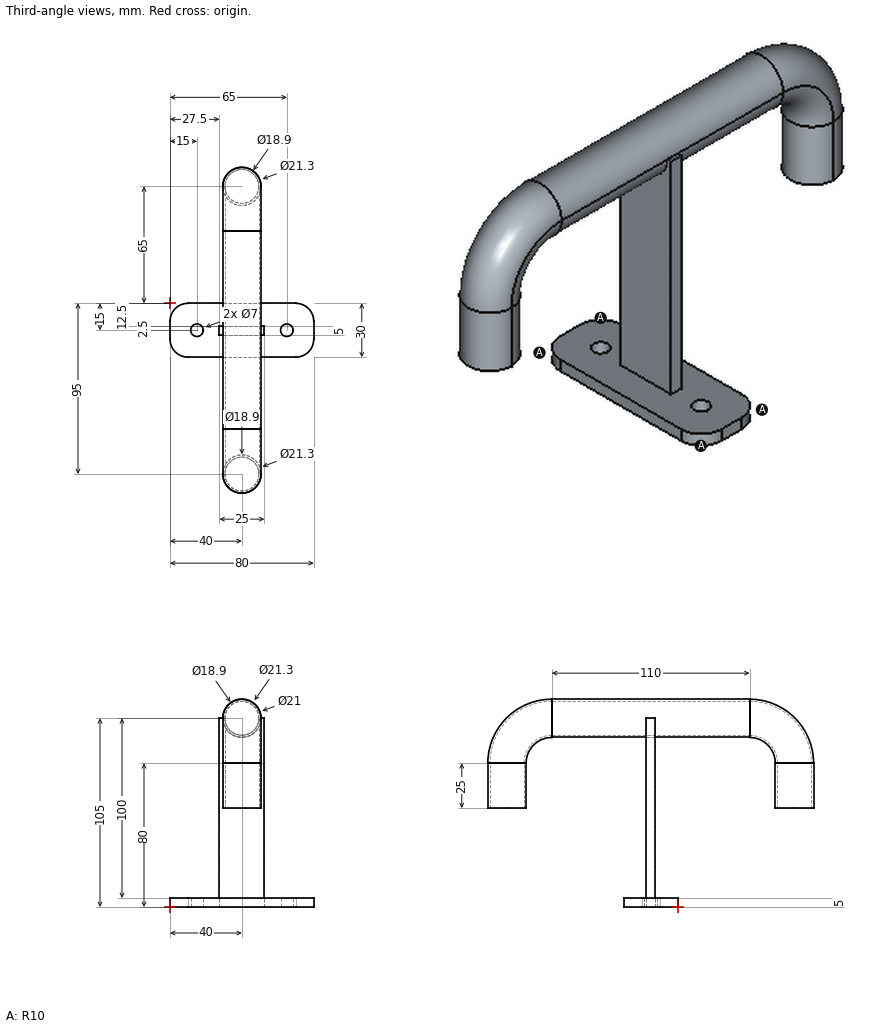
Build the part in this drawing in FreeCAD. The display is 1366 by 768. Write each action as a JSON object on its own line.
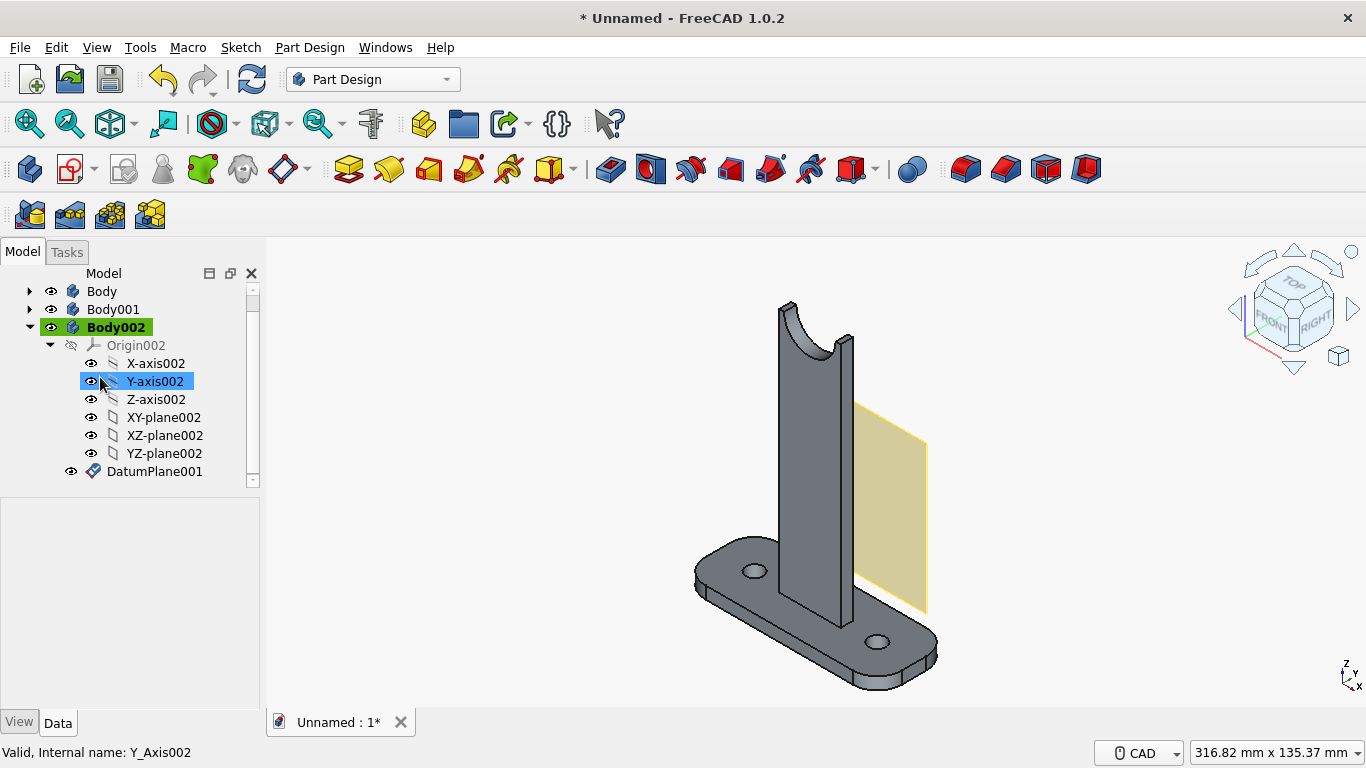
{"action": "left_click", "coordinate": [116, 471]}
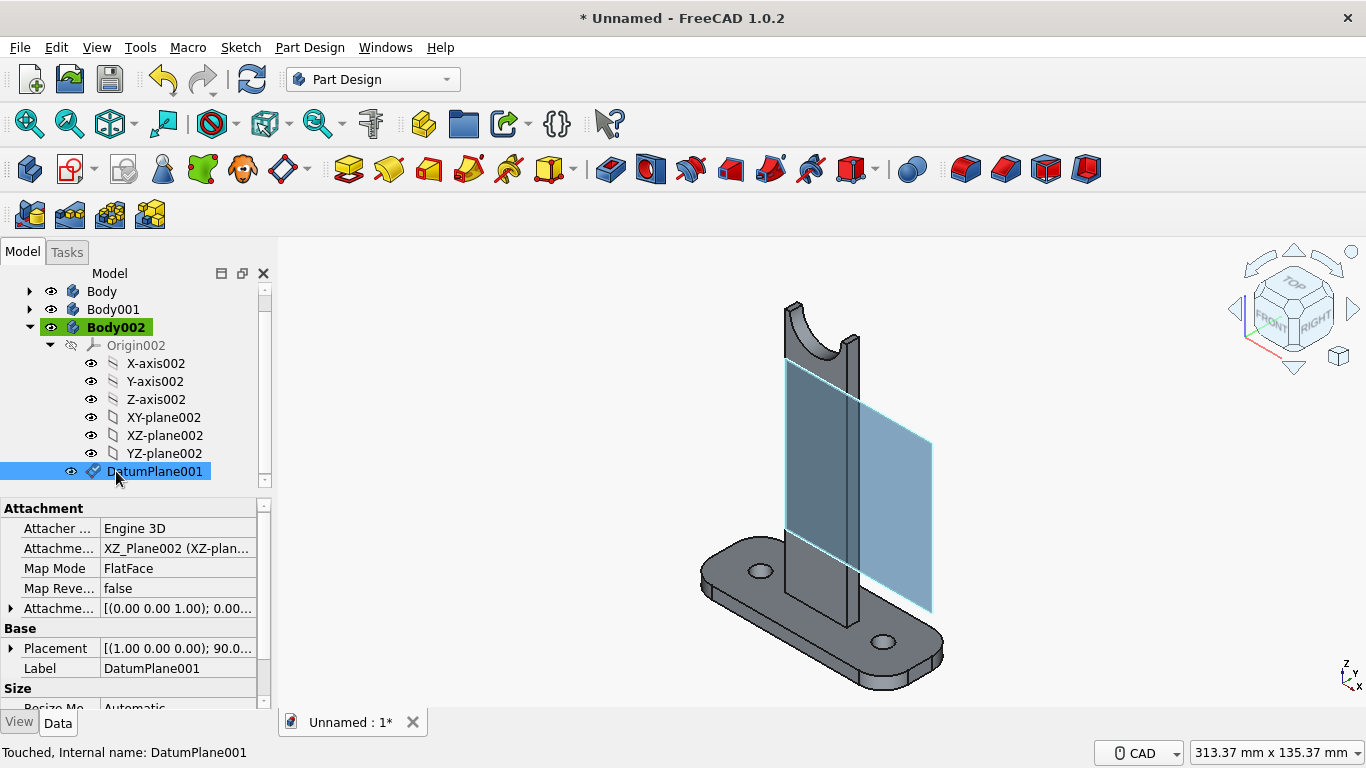
{"action": "left_click", "coordinate": [70, 170]}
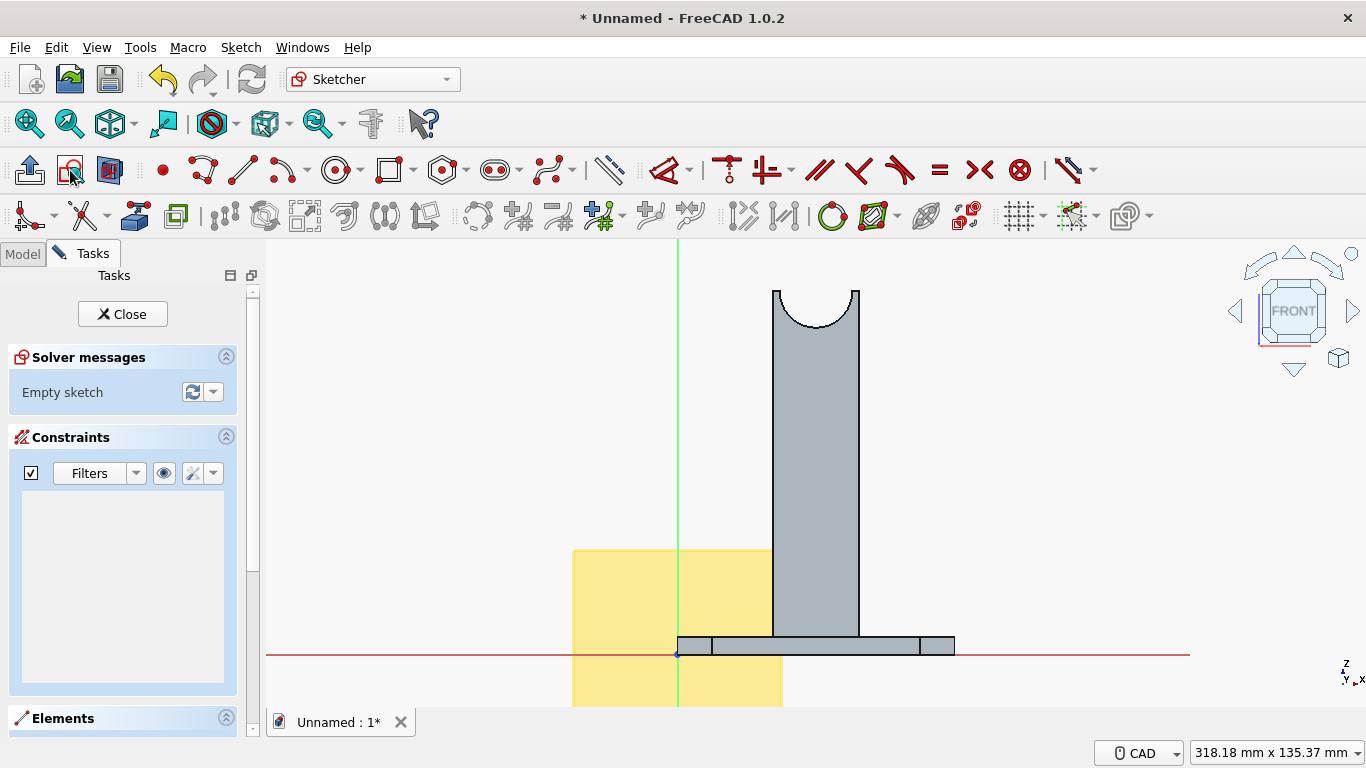
{"action": "scroll", "coordinate": [748, 473], "scroll_direction": "down", "scroll_amount": 5}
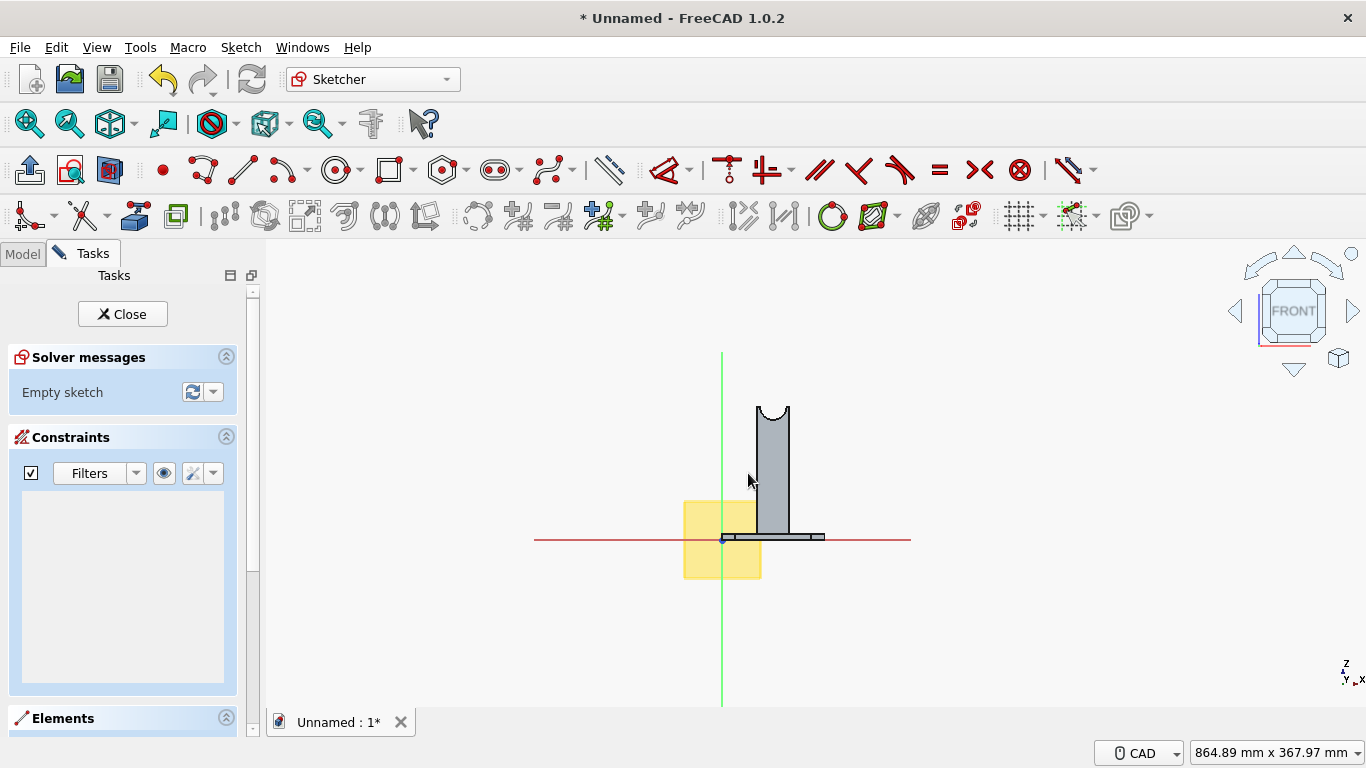
{"action": "scroll", "coordinate": [776, 400], "scroll_direction": "up", "scroll_amount": 12}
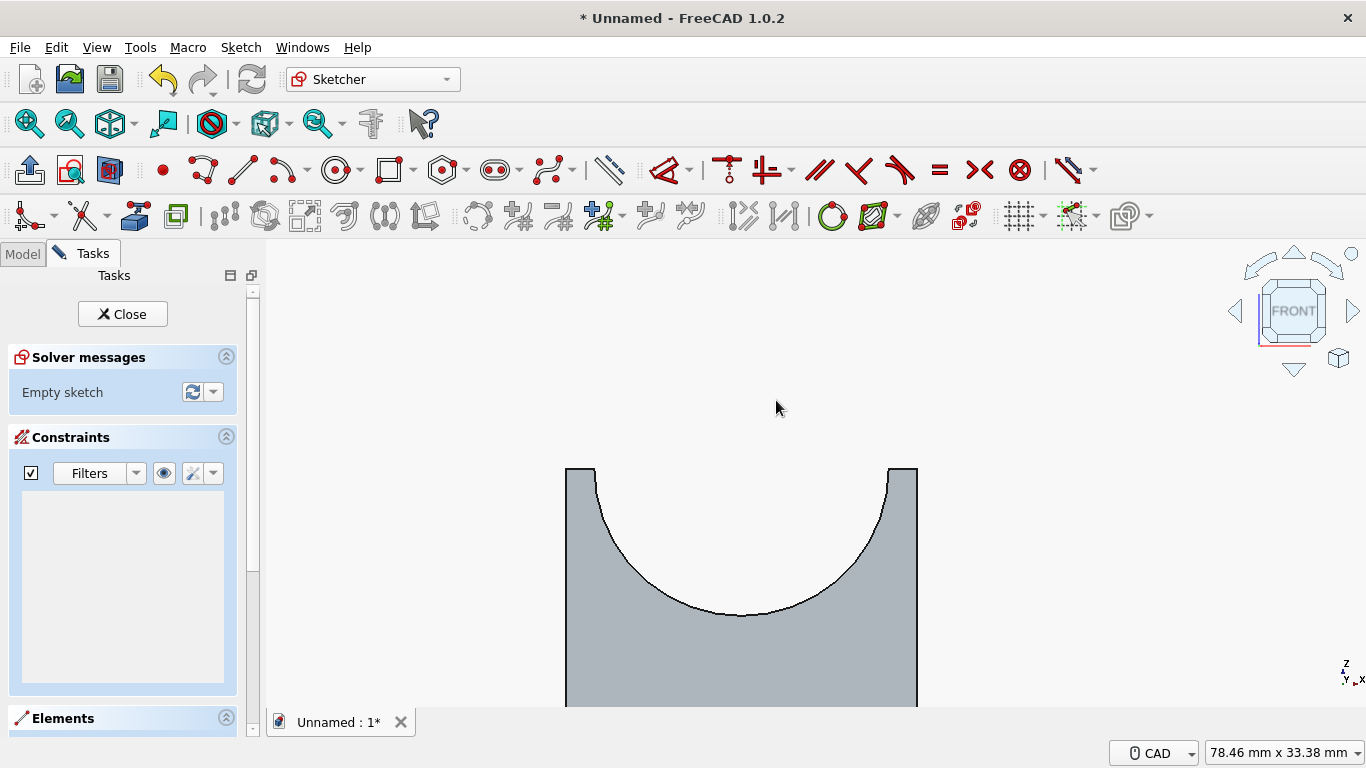
{"action": "left_click", "coordinate": [336, 170]}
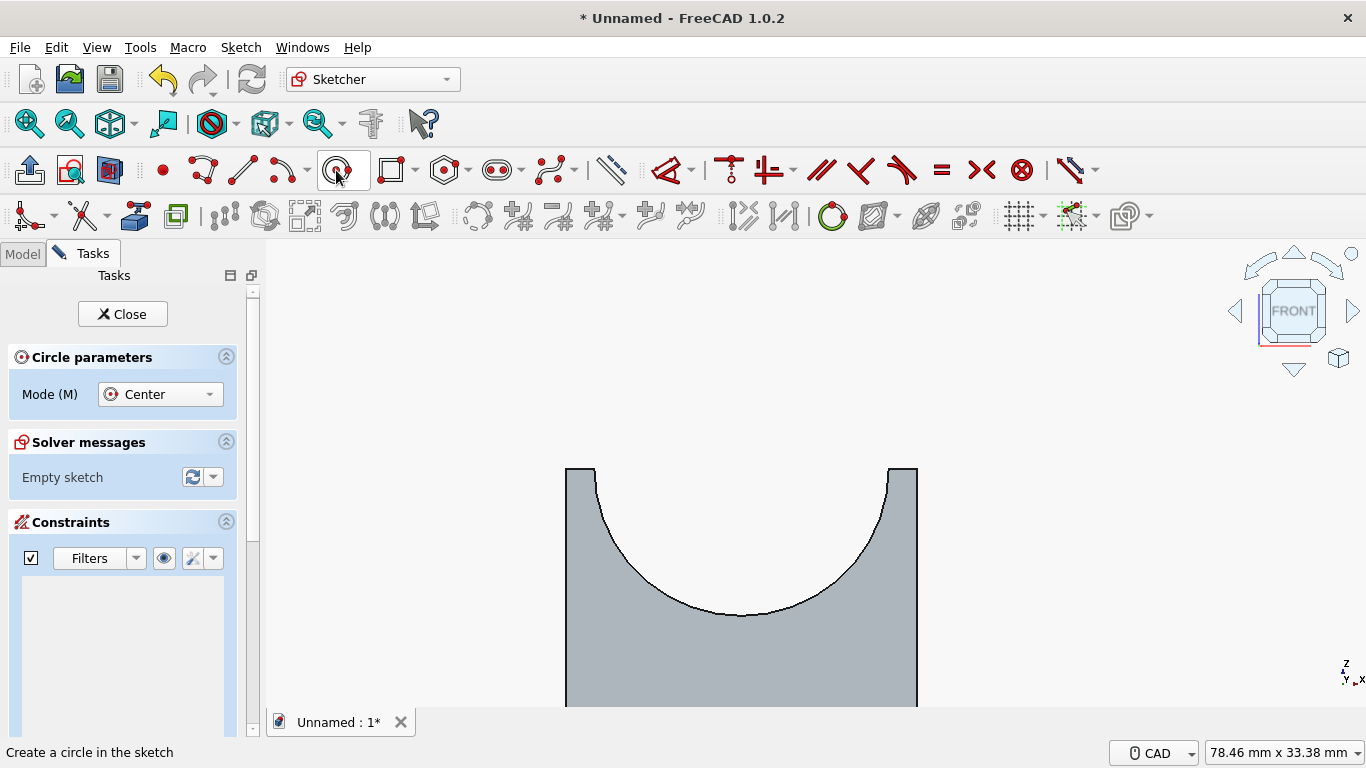
{"action": "left_click", "coordinate": [742, 469]}
{"action": "mouse_move", "coordinate": [847, 363]}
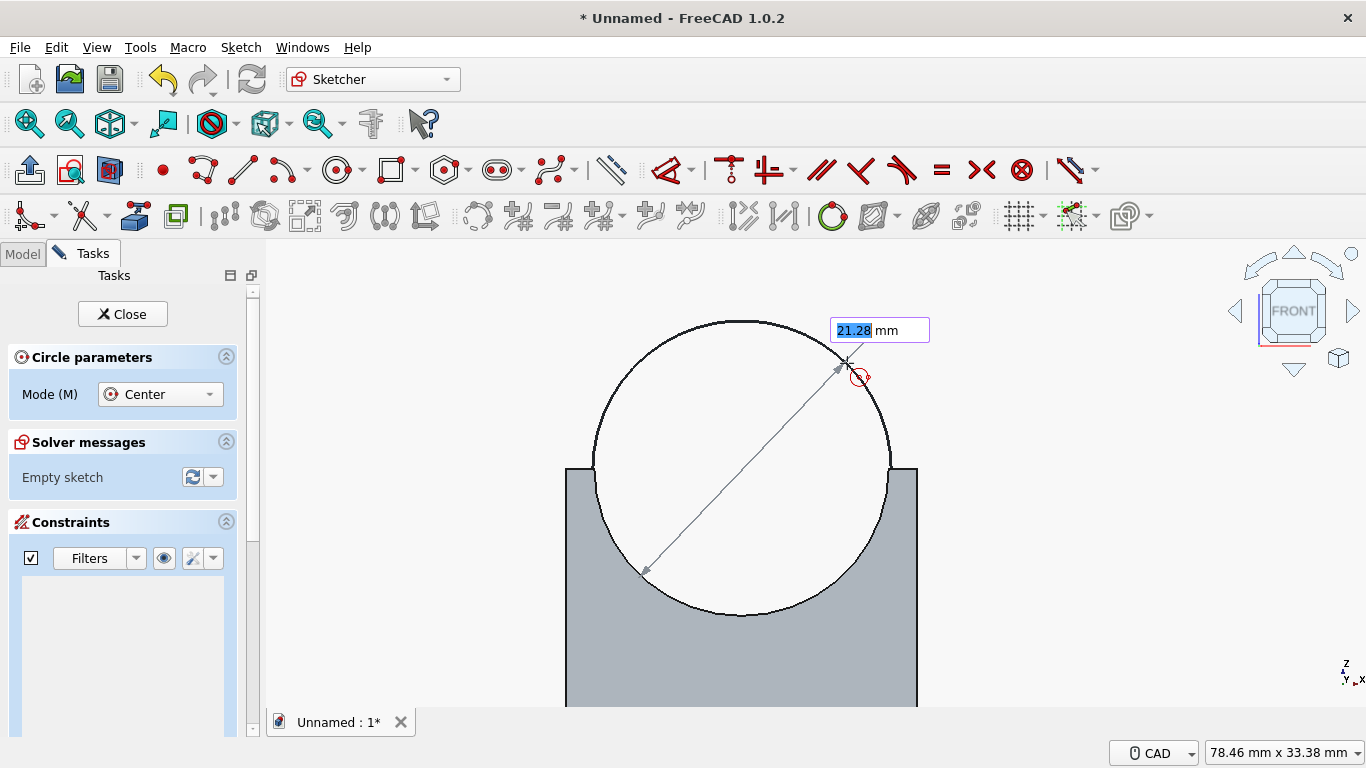
{"action": "type", "text": "21.3"}
{"action": "key", "text": "Return"}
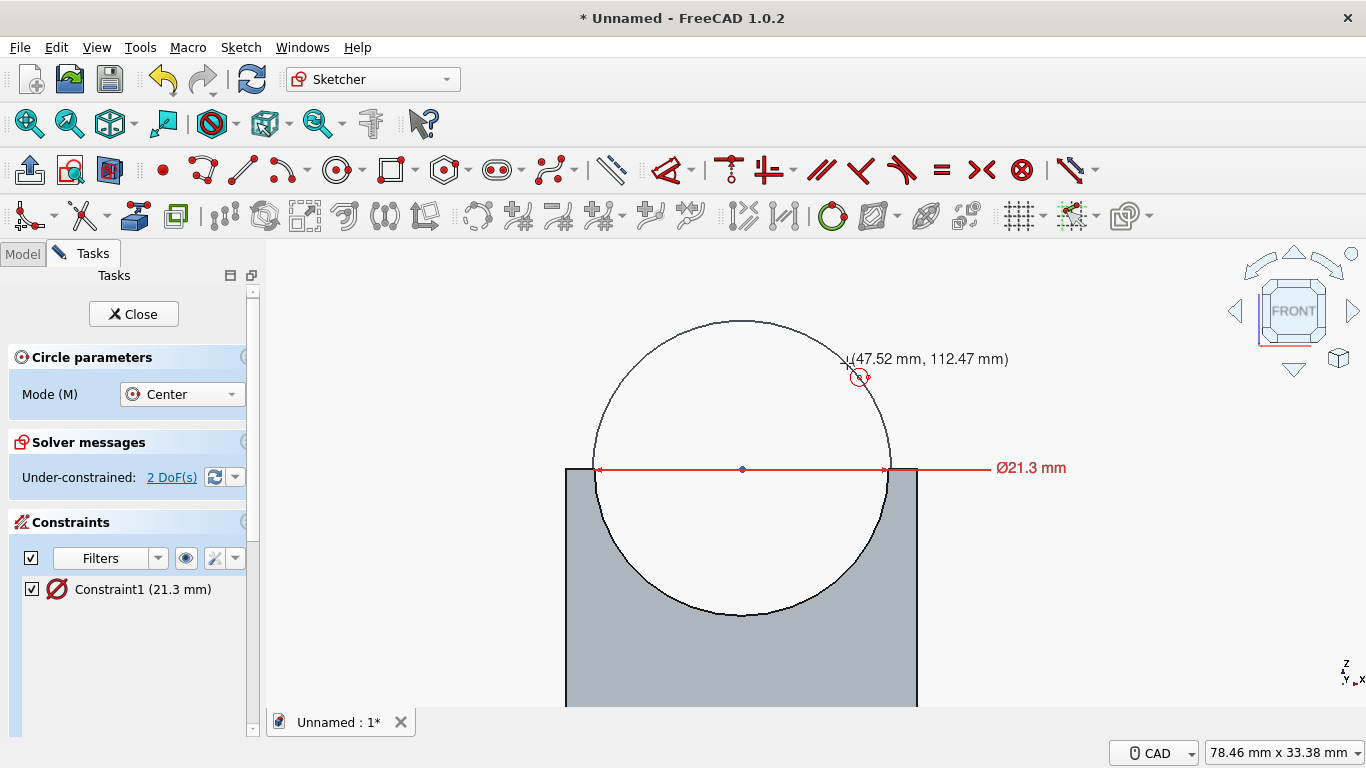
{"action": "left_click", "coordinate": [742, 470]}
{"action": "mouse_move", "coordinate": [835, 375]}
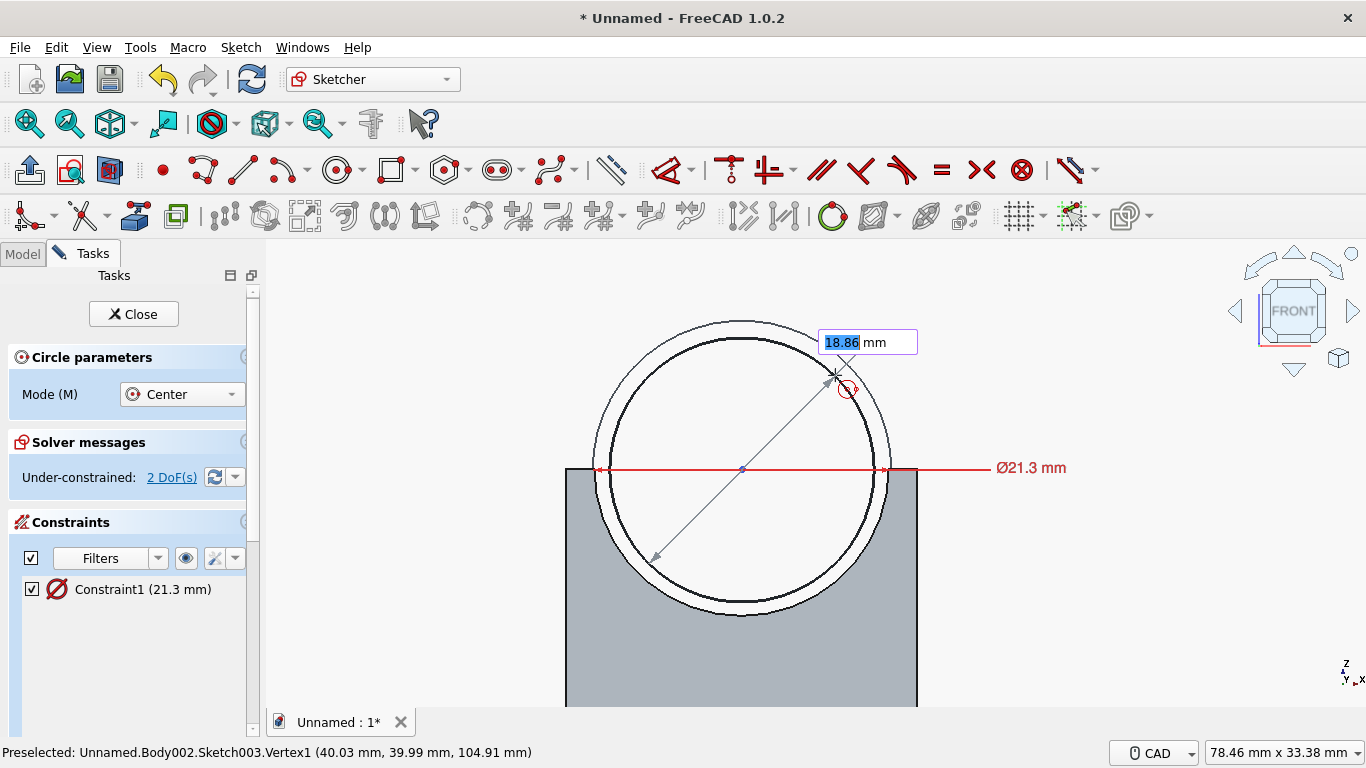
{"action": "type", "text": "18.9"}
{"action": "key", "text": "Return"}
{"action": "key", "text": "Escape"}